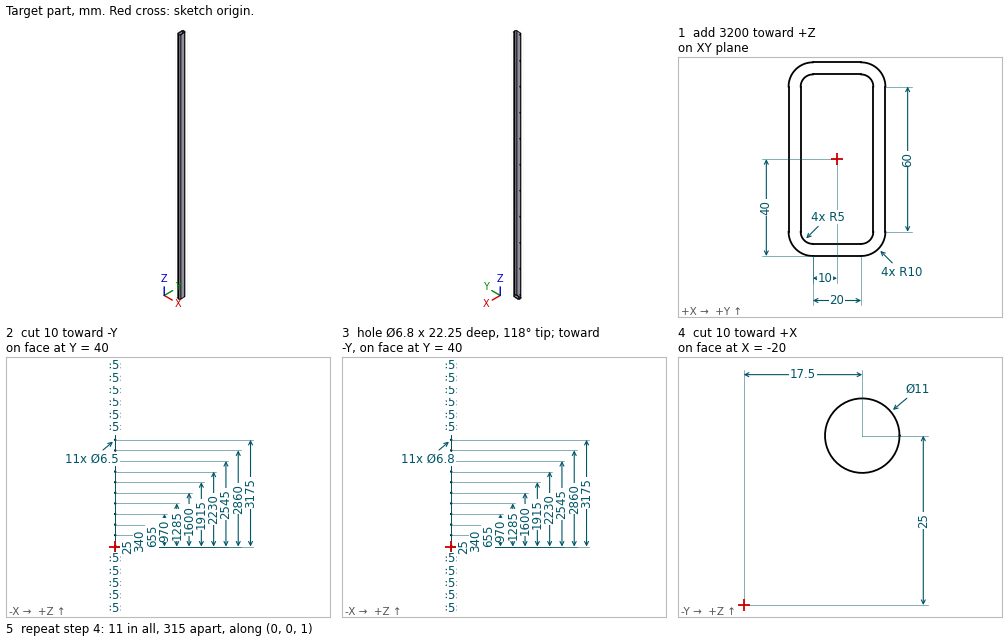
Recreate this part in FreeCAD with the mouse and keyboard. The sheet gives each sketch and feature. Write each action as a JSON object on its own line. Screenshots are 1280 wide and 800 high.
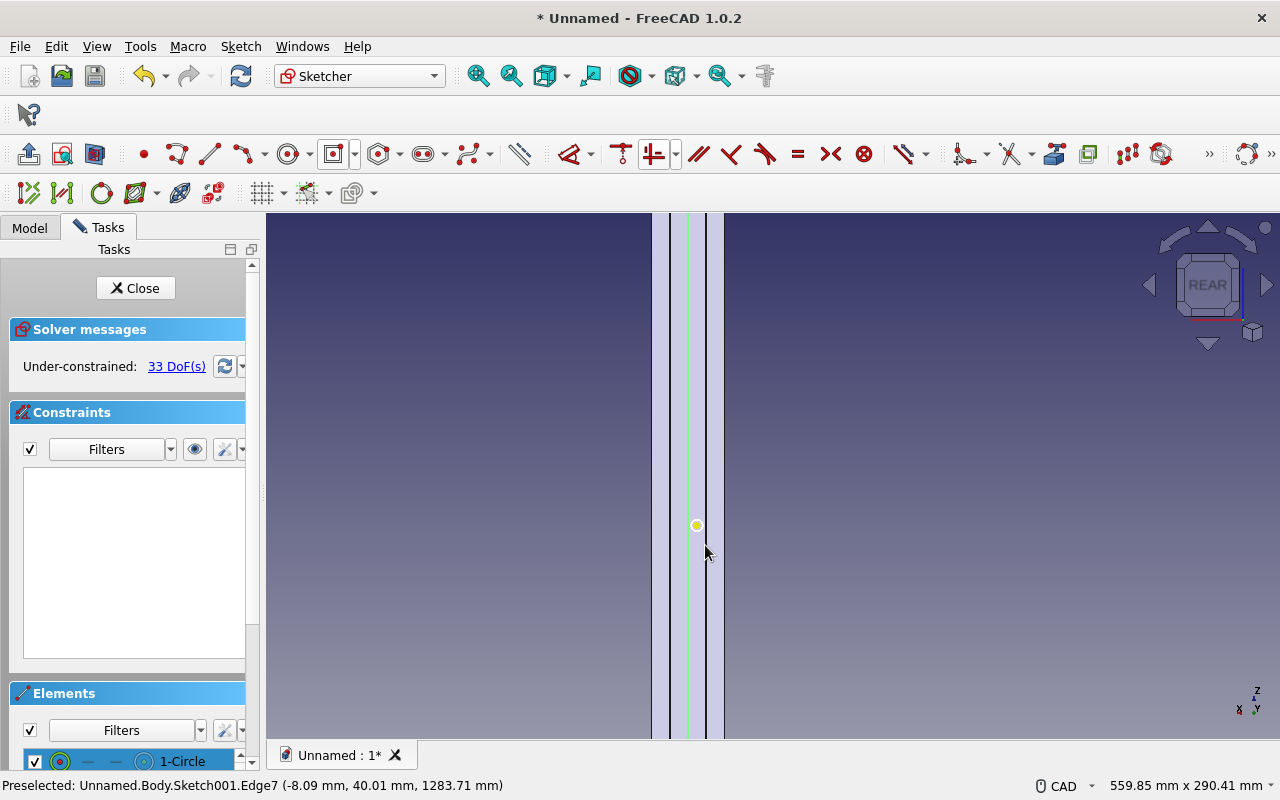
{"action": "left_click", "coordinate": [701, 530]}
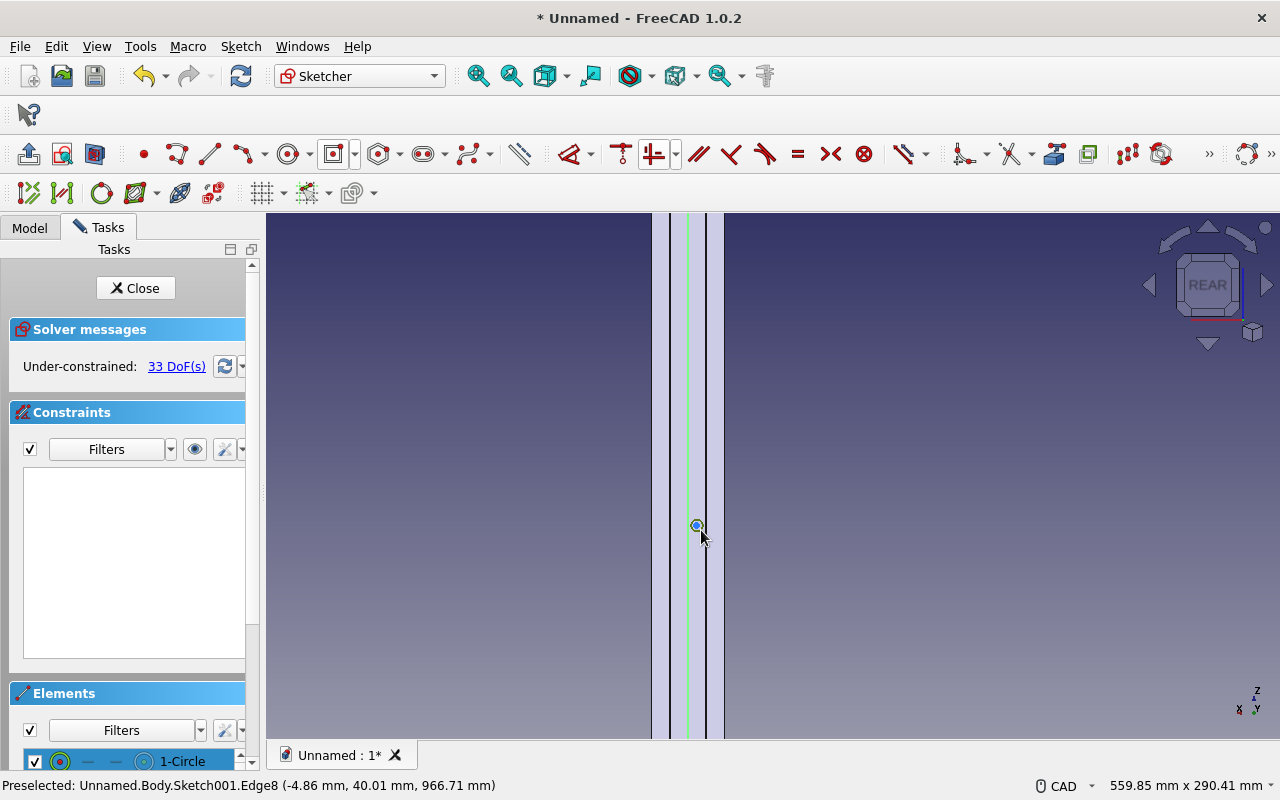
{"action": "scroll", "coordinate": [705, 545], "scroll_direction": "down", "scroll_amount": 14}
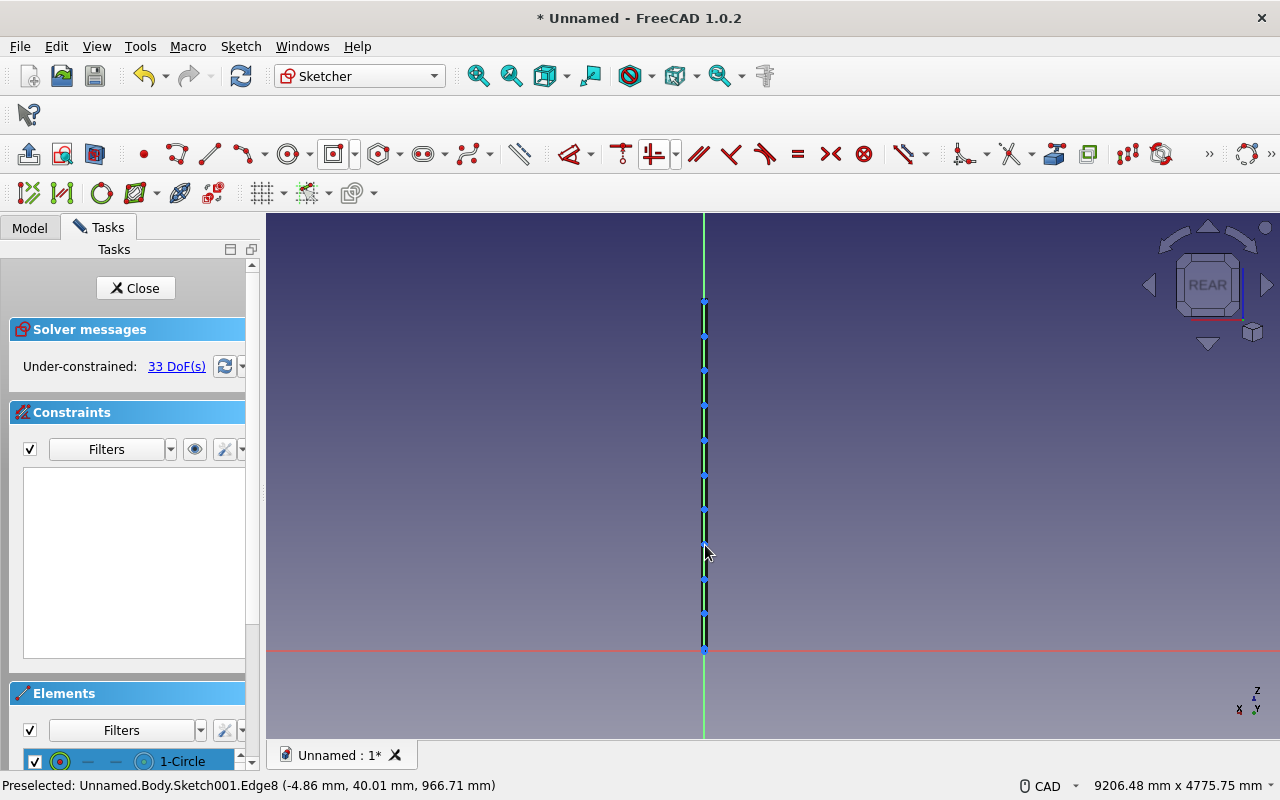
{"action": "scroll", "coordinate": [705, 579], "scroll_direction": "up", "scroll_amount": 14}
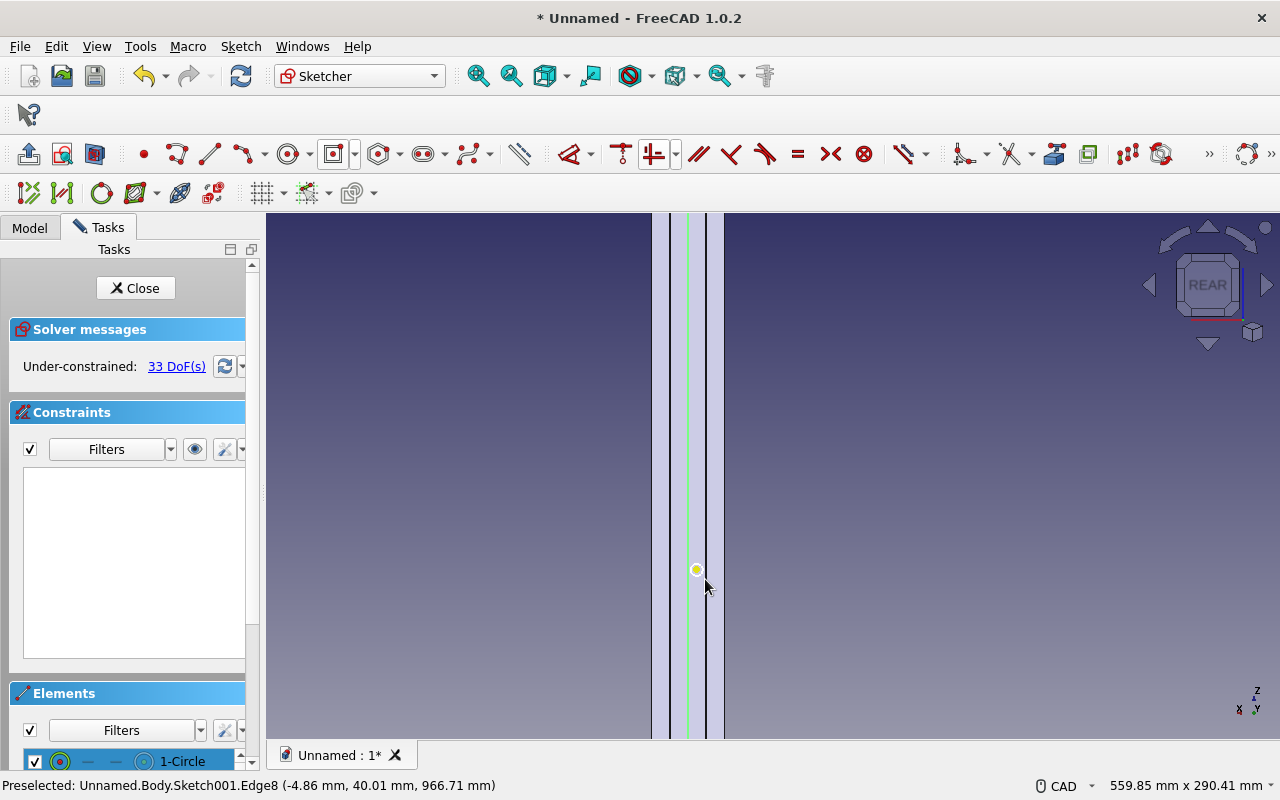
{"action": "left_click", "coordinate": [701, 574]}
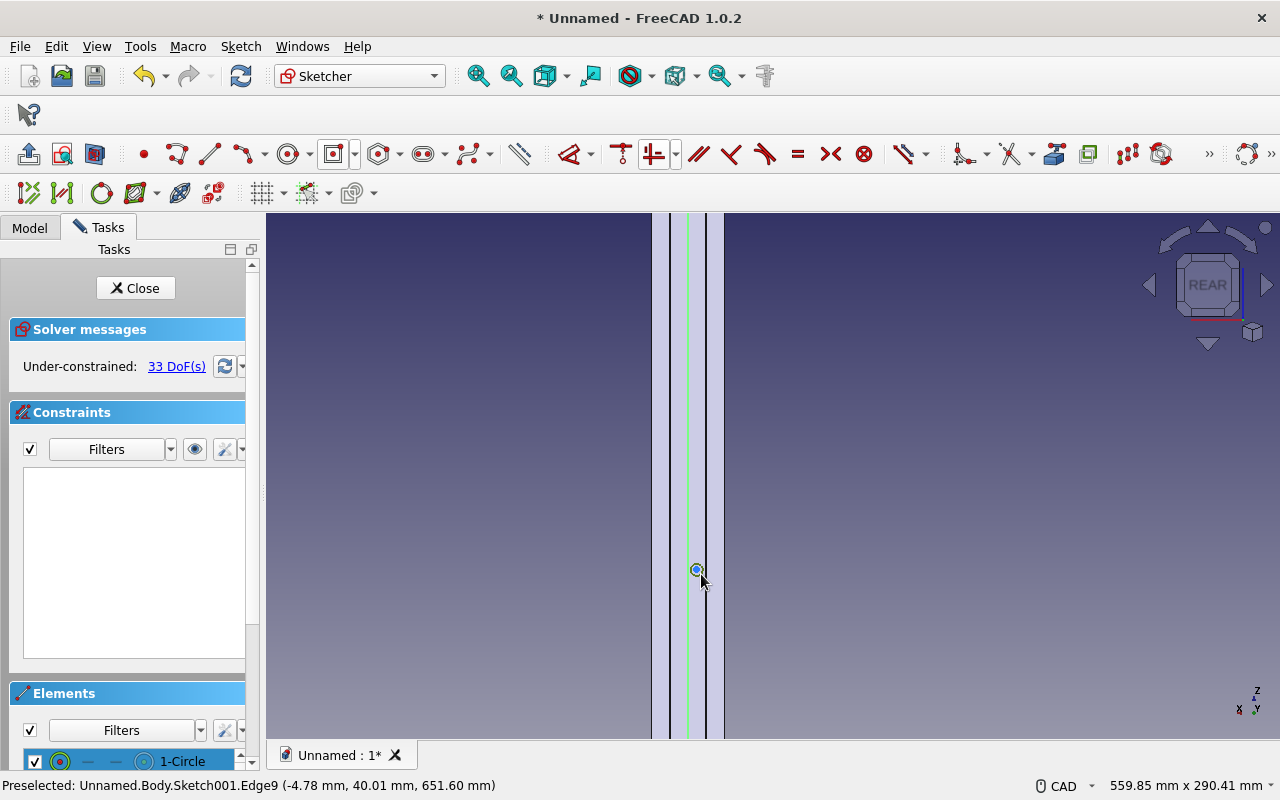
{"action": "scroll", "coordinate": [705, 579], "scroll_direction": "down", "scroll_amount": 14}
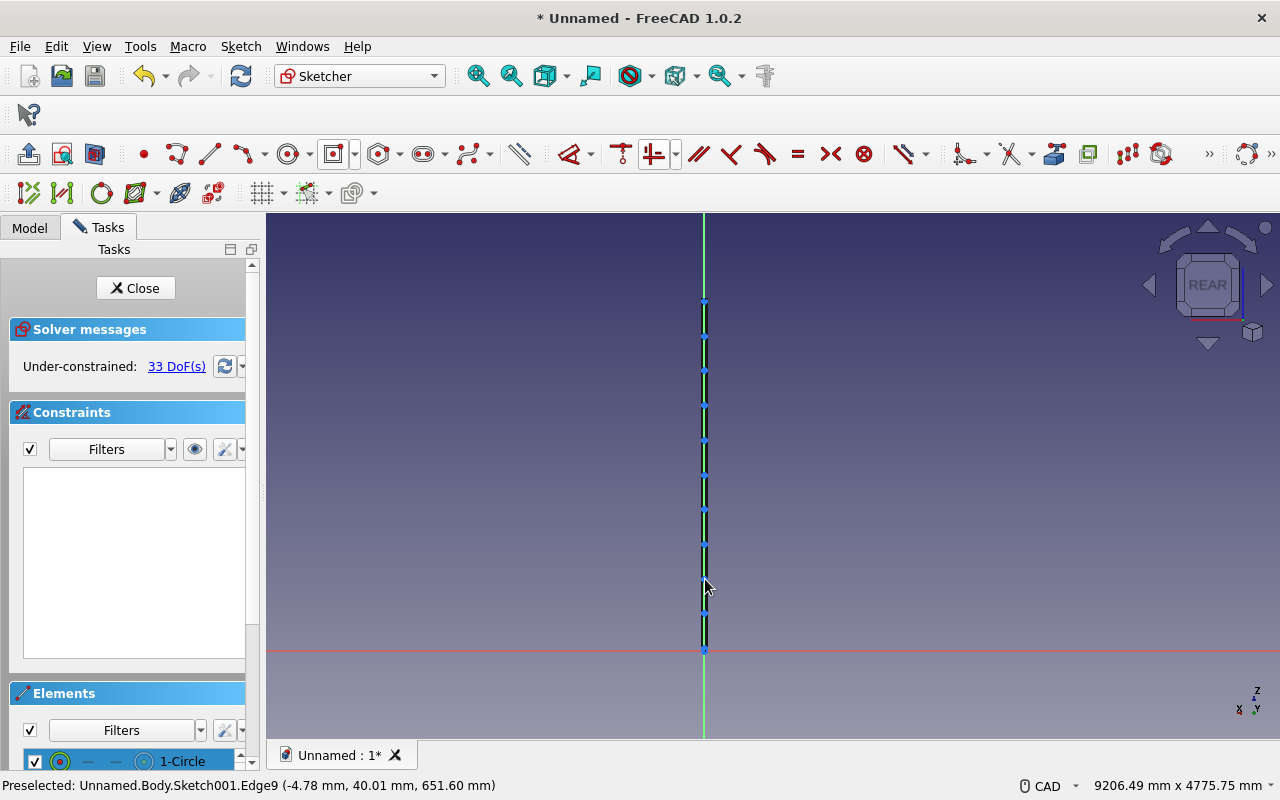
{"action": "scroll", "coordinate": [705, 614], "scroll_direction": "up", "scroll_amount": 14}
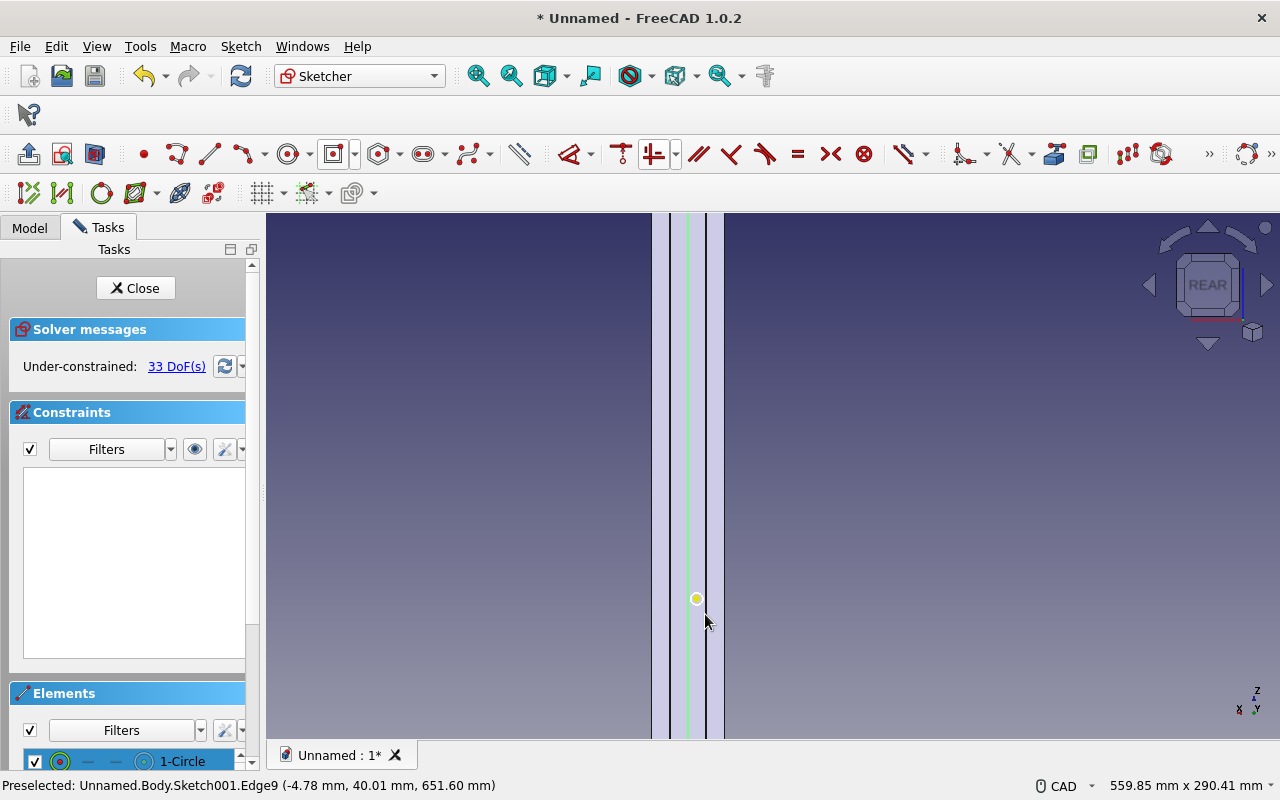
{"action": "left_click", "coordinate": [701, 595]}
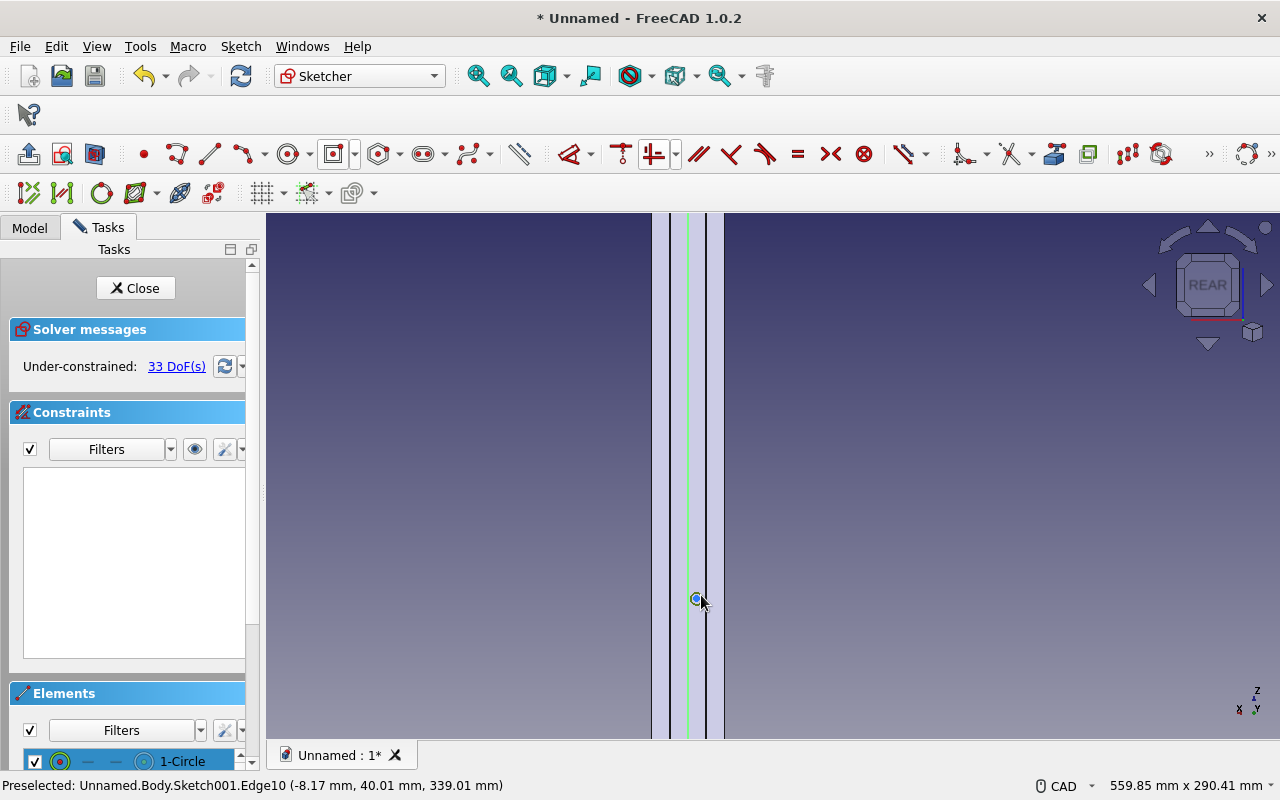
{"action": "scroll", "coordinate": [705, 615], "scroll_direction": "down", "scroll_amount": 14}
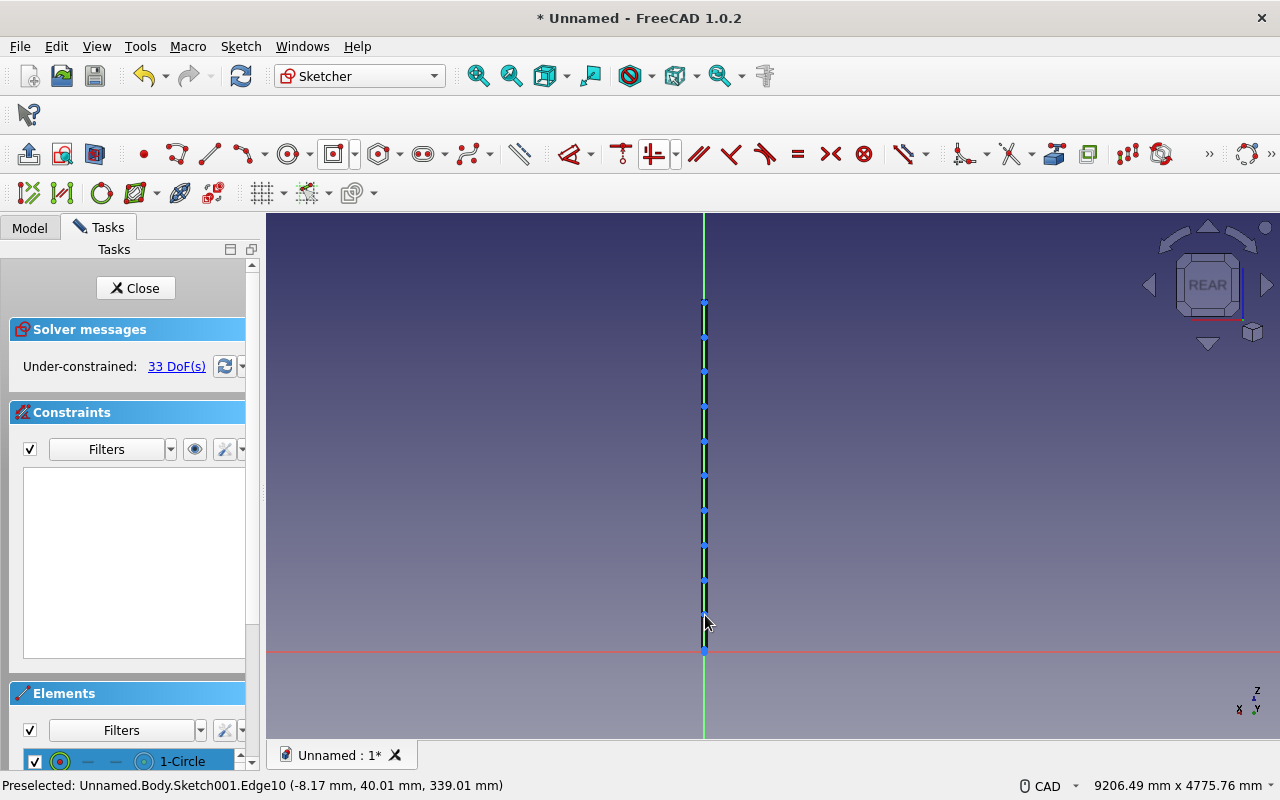
{"action": "scroll", "coordinate": [705, 650], "scroll_direction": "up", "scroll_amount": 14}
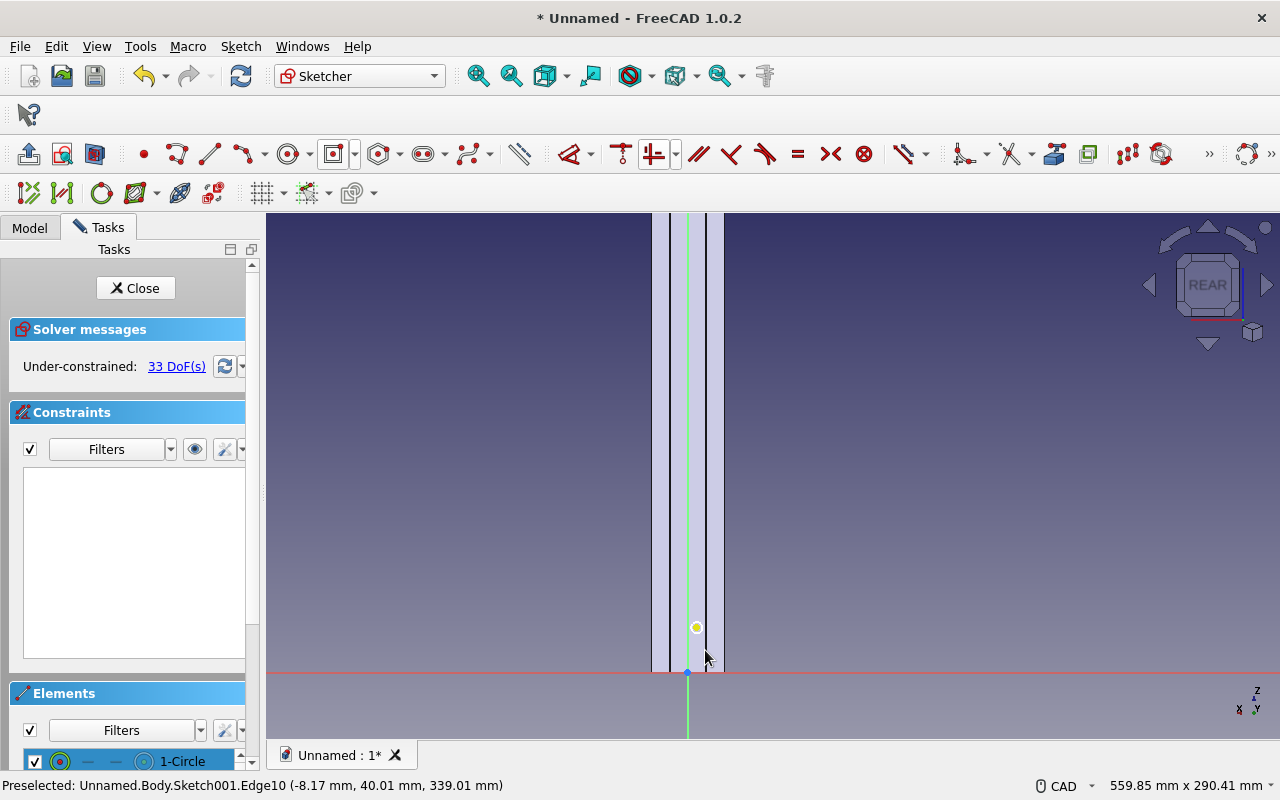
{"action": "left_click", "coordinate": [701, 632]}